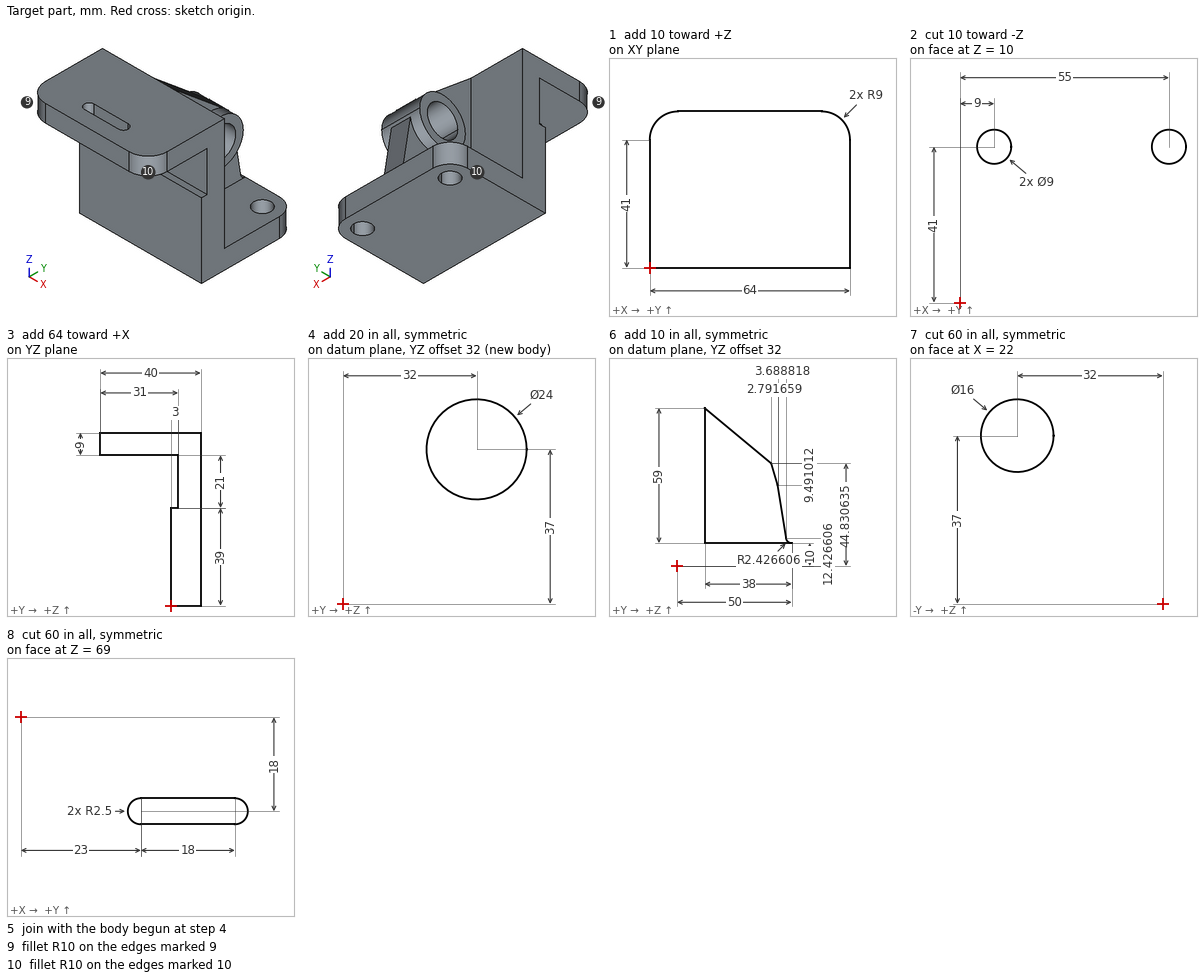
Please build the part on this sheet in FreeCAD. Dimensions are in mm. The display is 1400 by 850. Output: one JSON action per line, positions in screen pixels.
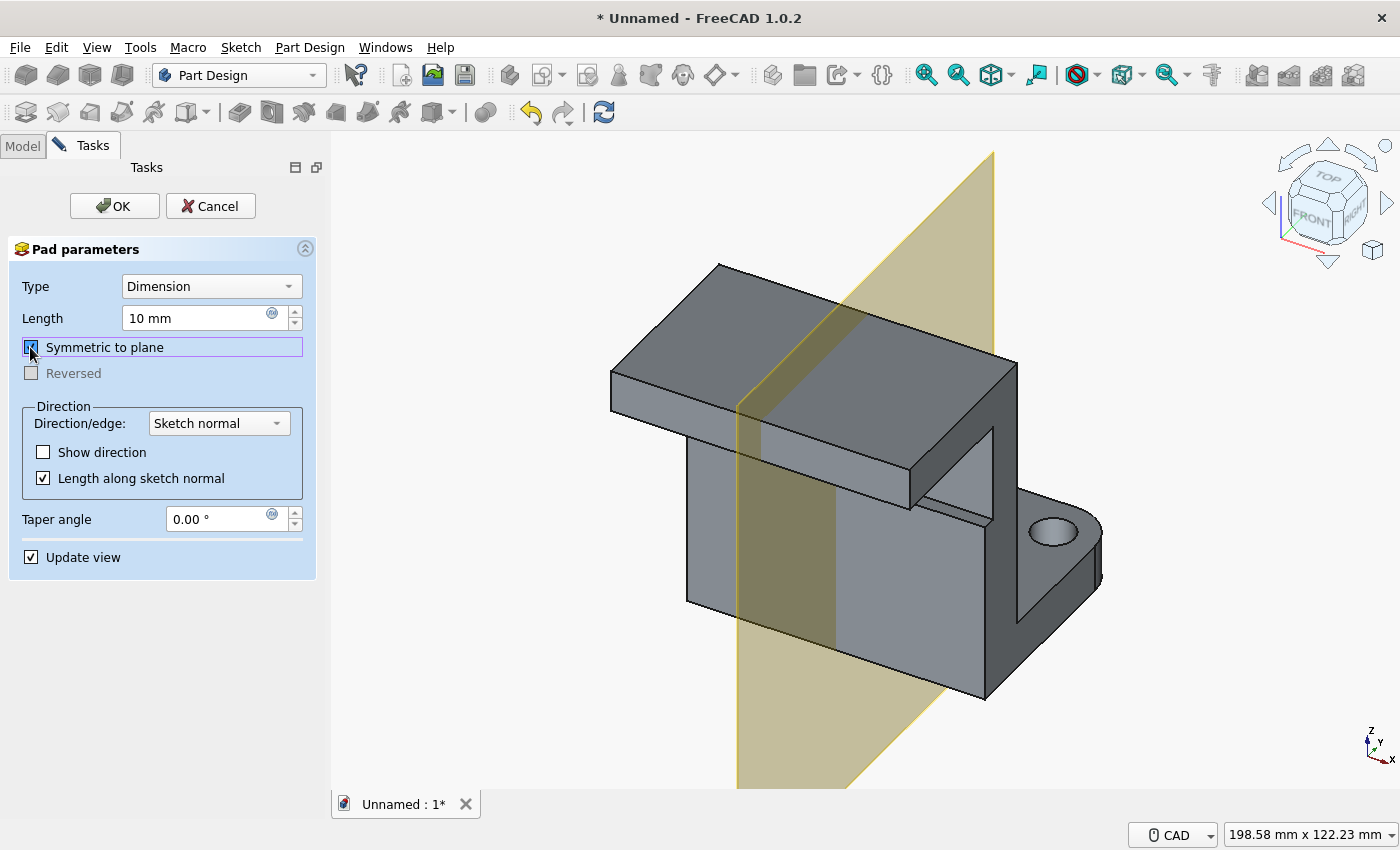
{"action": "left_click", "coordinate": [115, 206]}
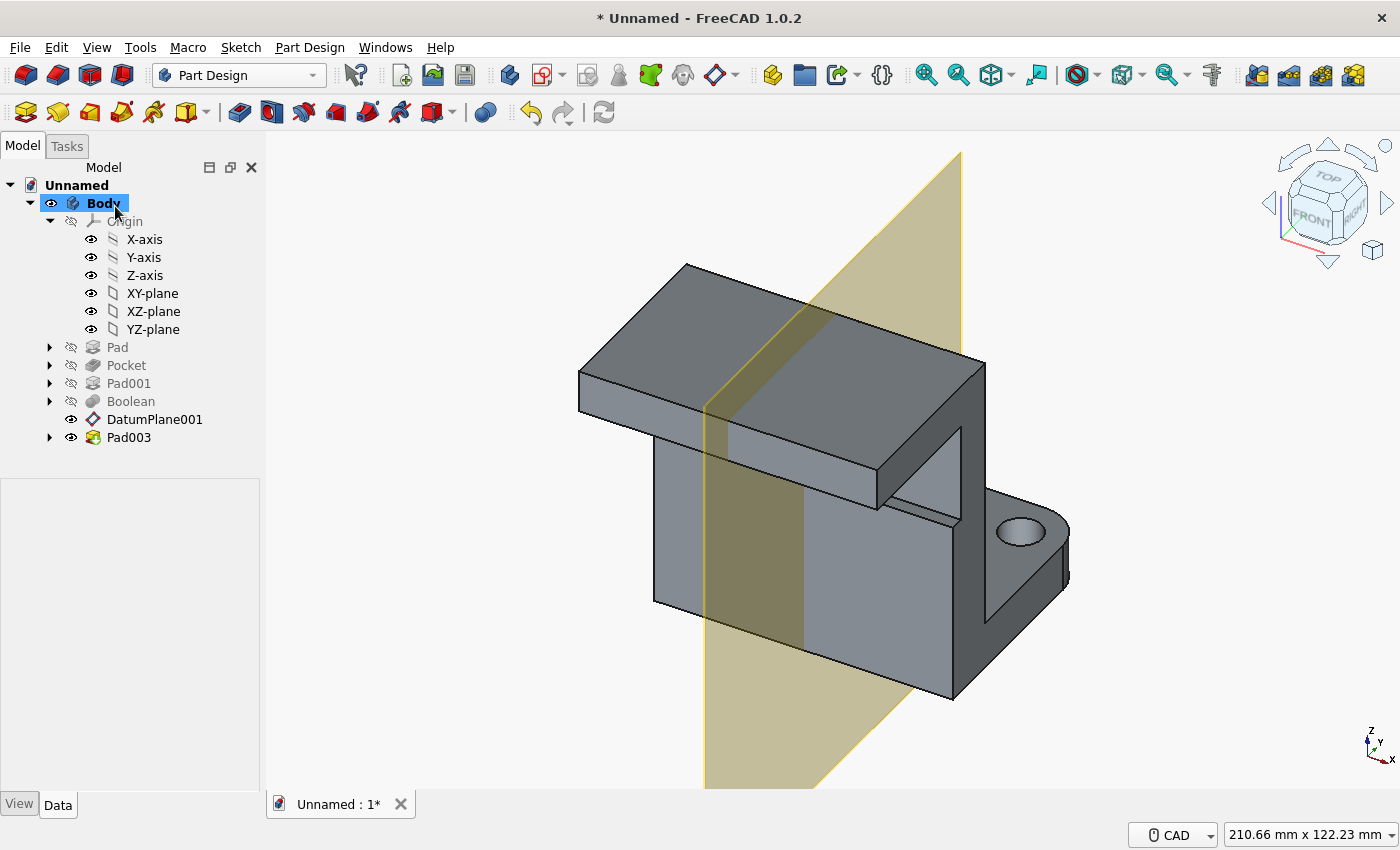
{"action": "left_click", "coordinate": [116, 419]}
{"action": "key", "text": "space"}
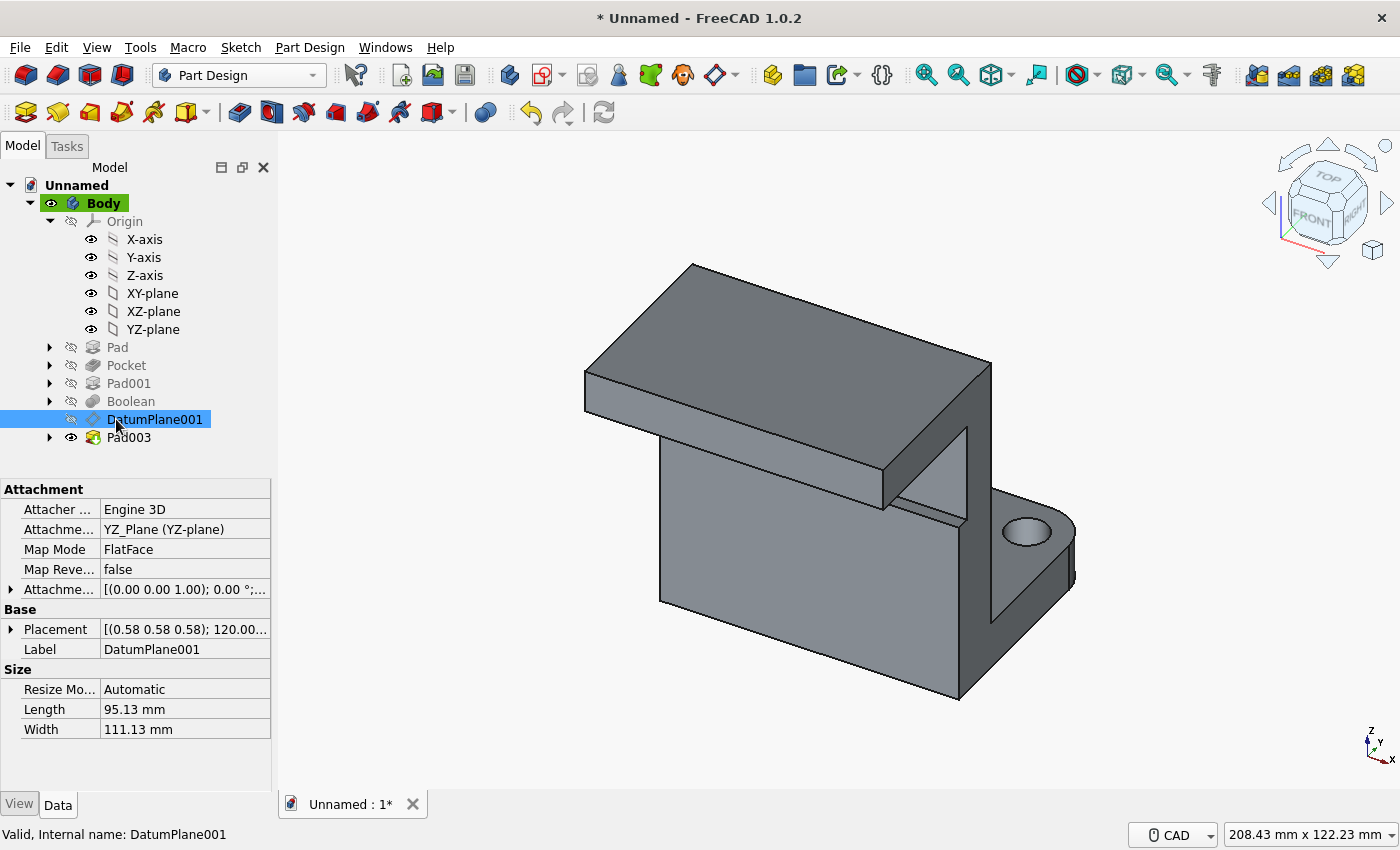
{"action": "key", "text": "6"}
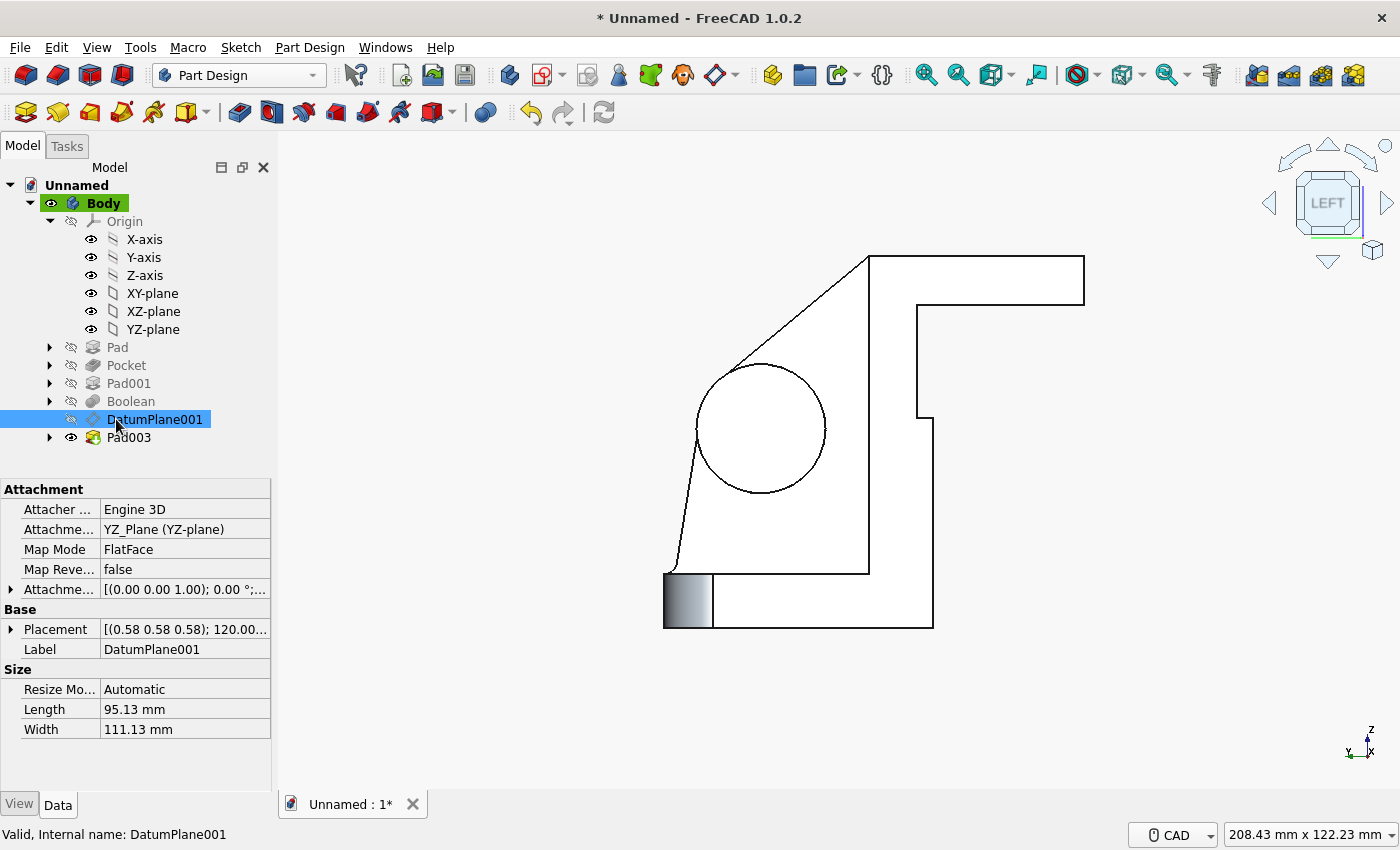
{"action": "left_click", "coordinate": [761, 428]}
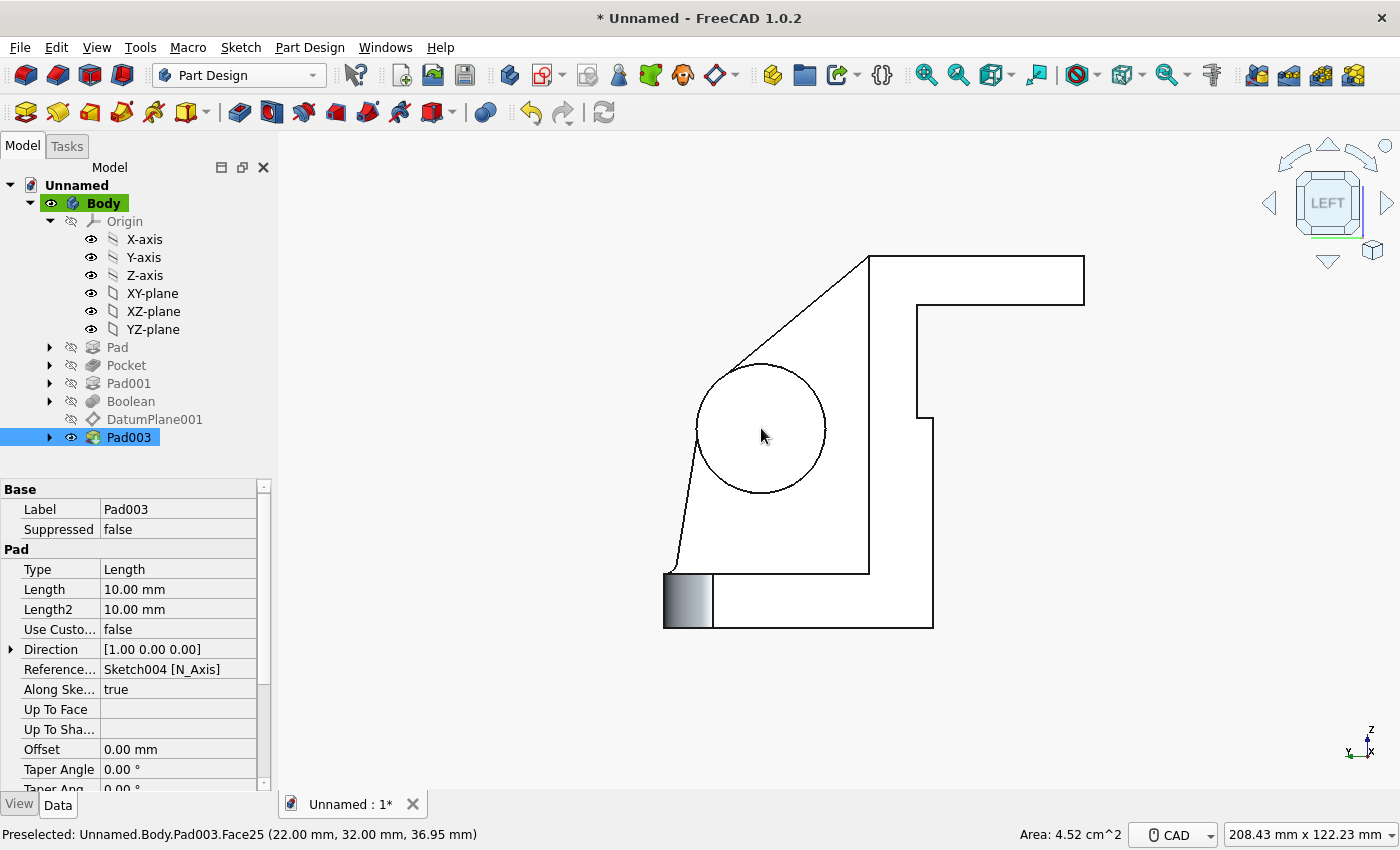
{"action": "left_click", "coordinate": [542, 76]}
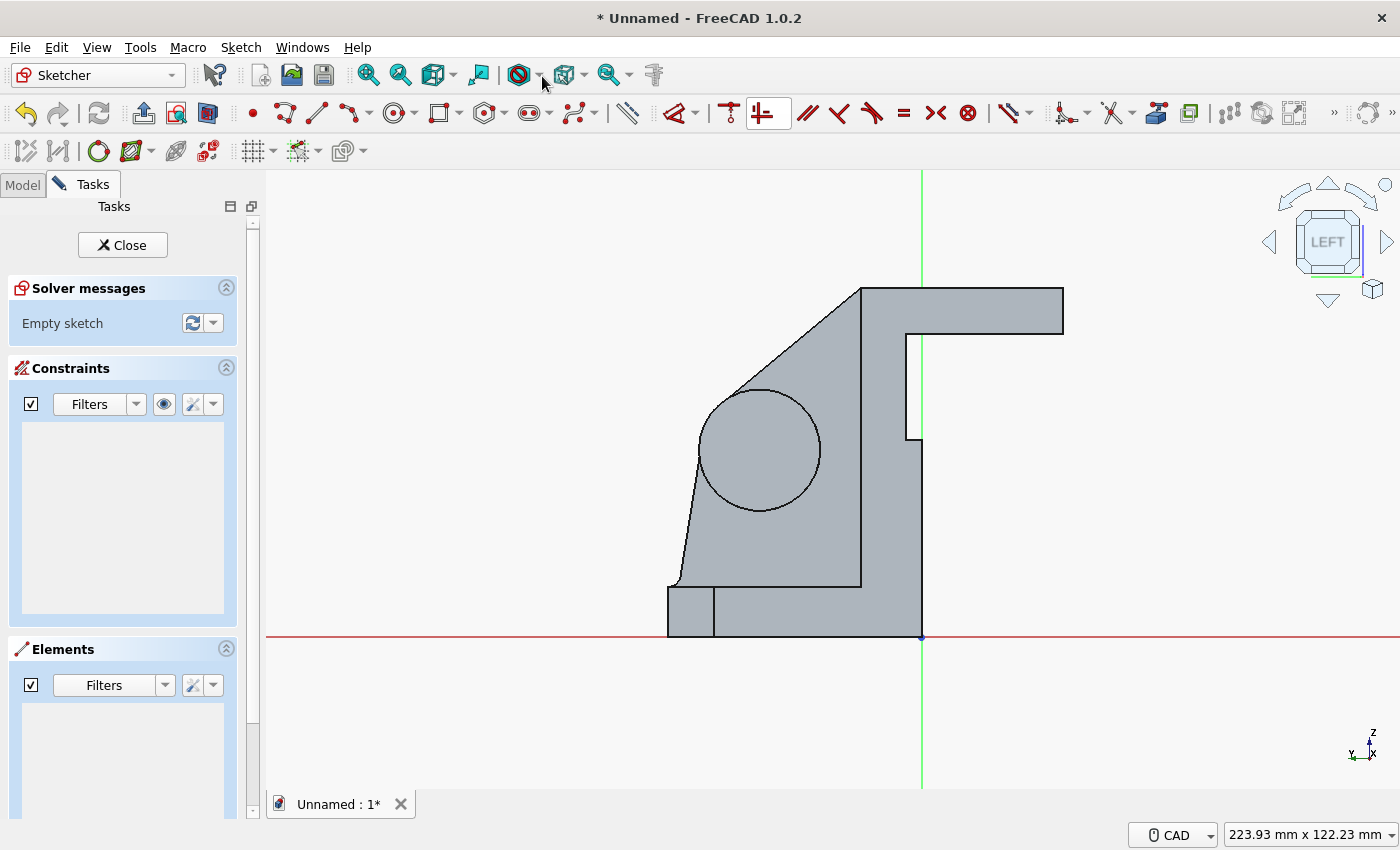
{"action": "scroll", "coordinate": [758, 443], "scroll_direction": "up", "scroll_amount": 8}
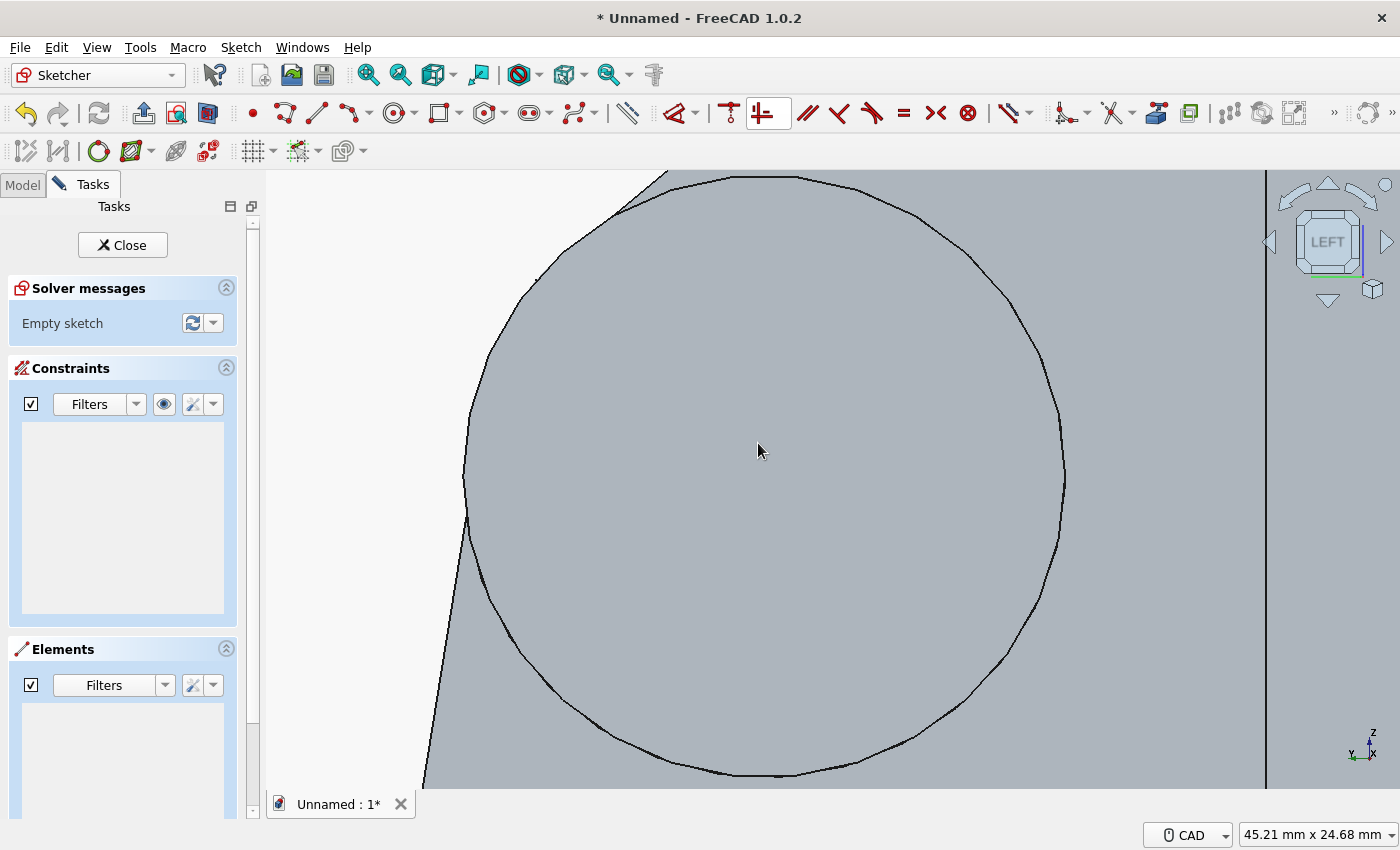
{"action": "left_click", "coordinate": [394, 114]}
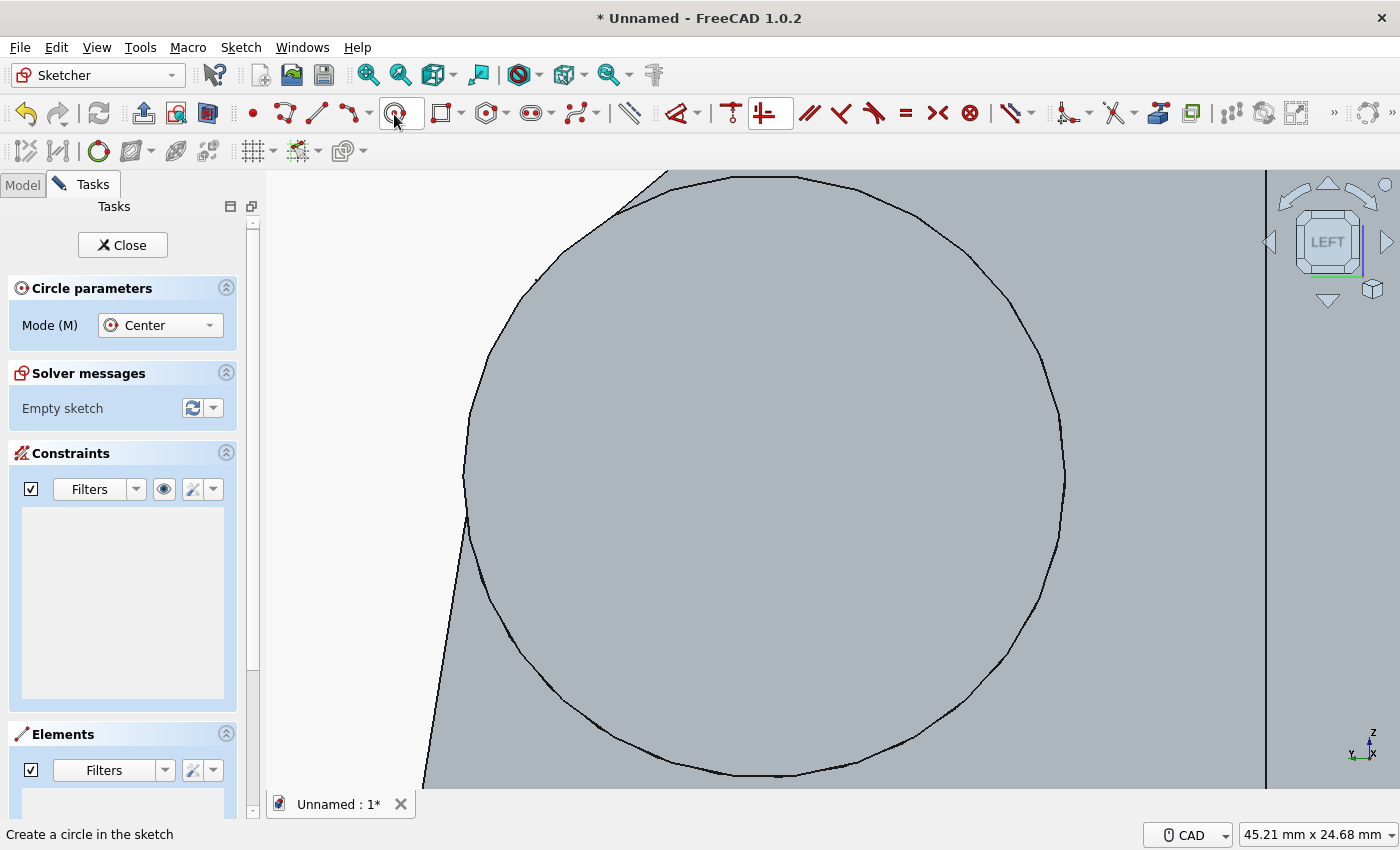
{"action": "left_click", "coordinate": [764, 476]}
{"action": "mouse_move", "coordinate": [906, 334]}